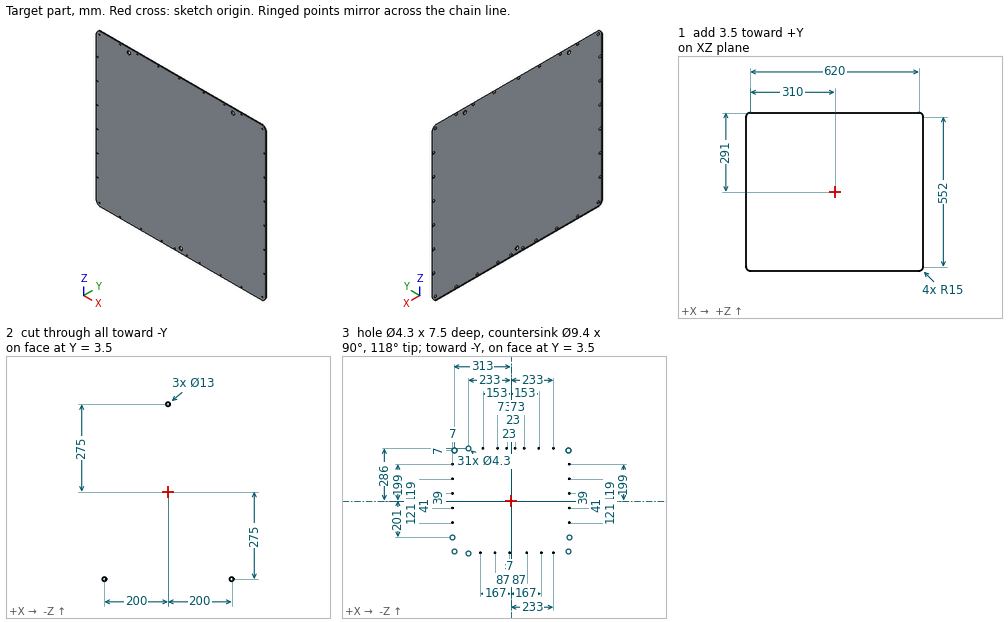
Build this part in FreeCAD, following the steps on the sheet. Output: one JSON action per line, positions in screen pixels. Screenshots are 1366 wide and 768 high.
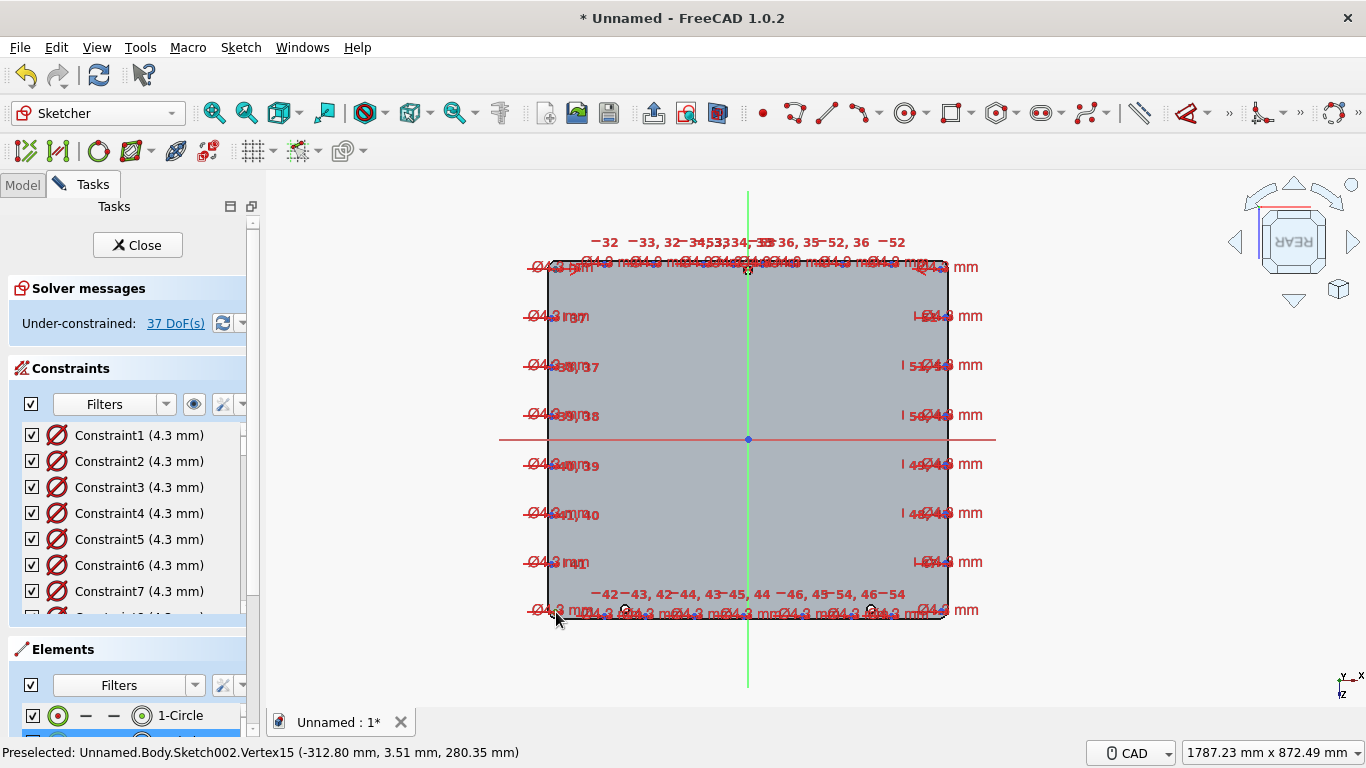
{"action": "left_click", "coordinate": [618, 440]}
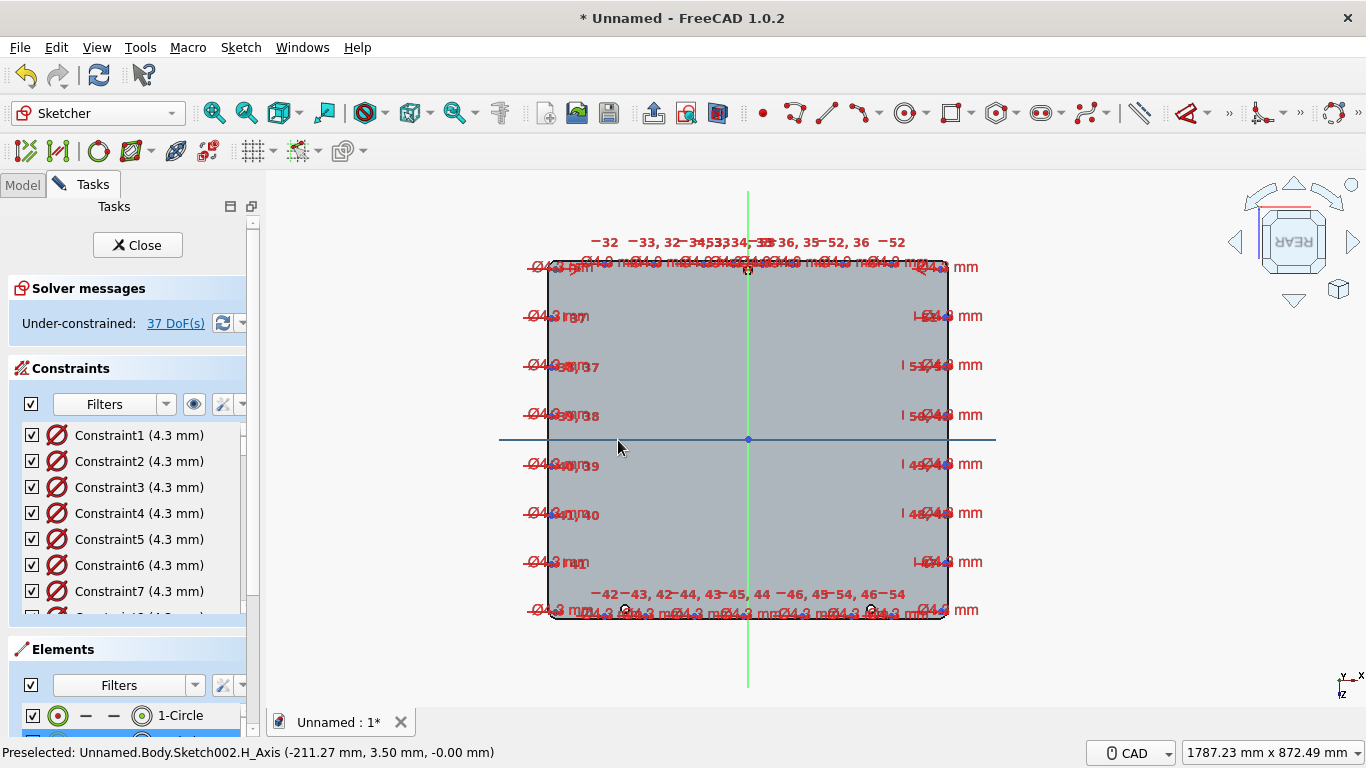
{"action": "key", "text": "s"}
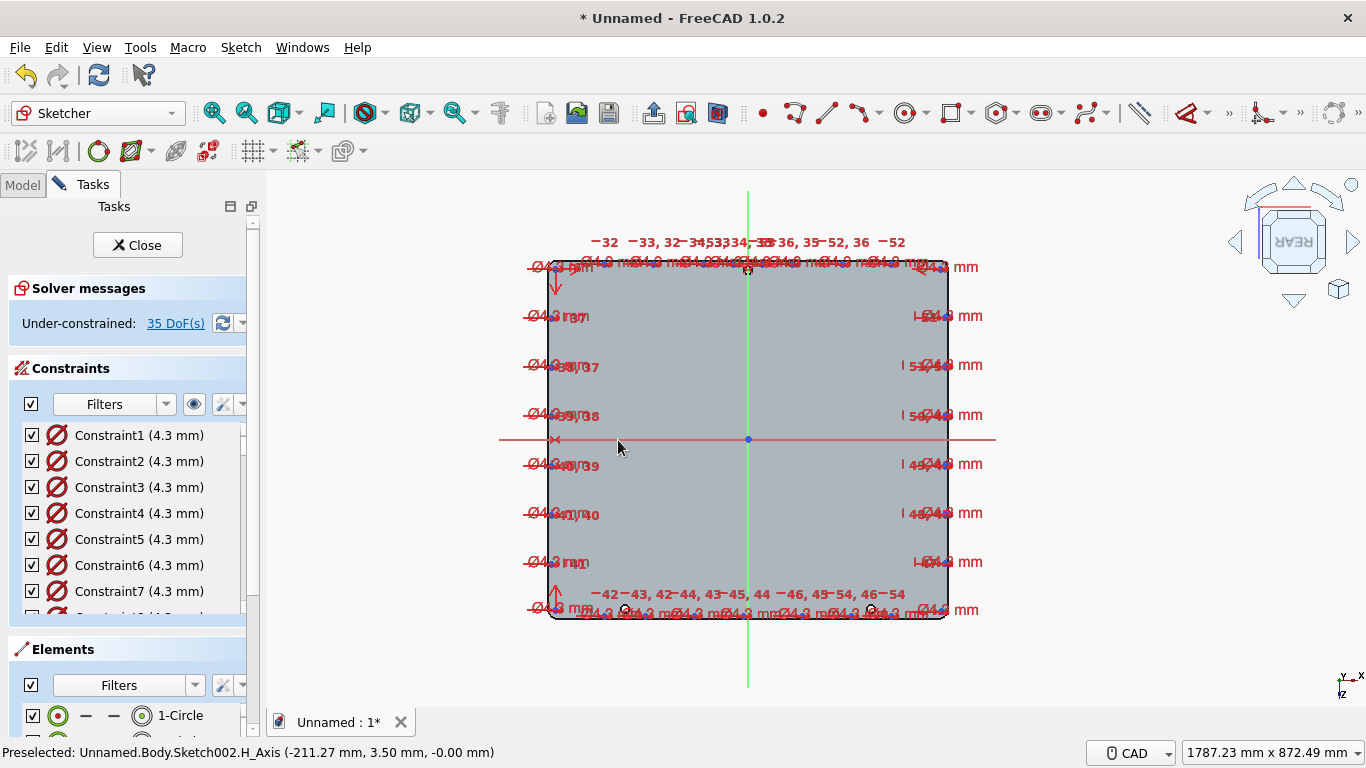
{"action": "left_click", "coordinate": [605, 264]}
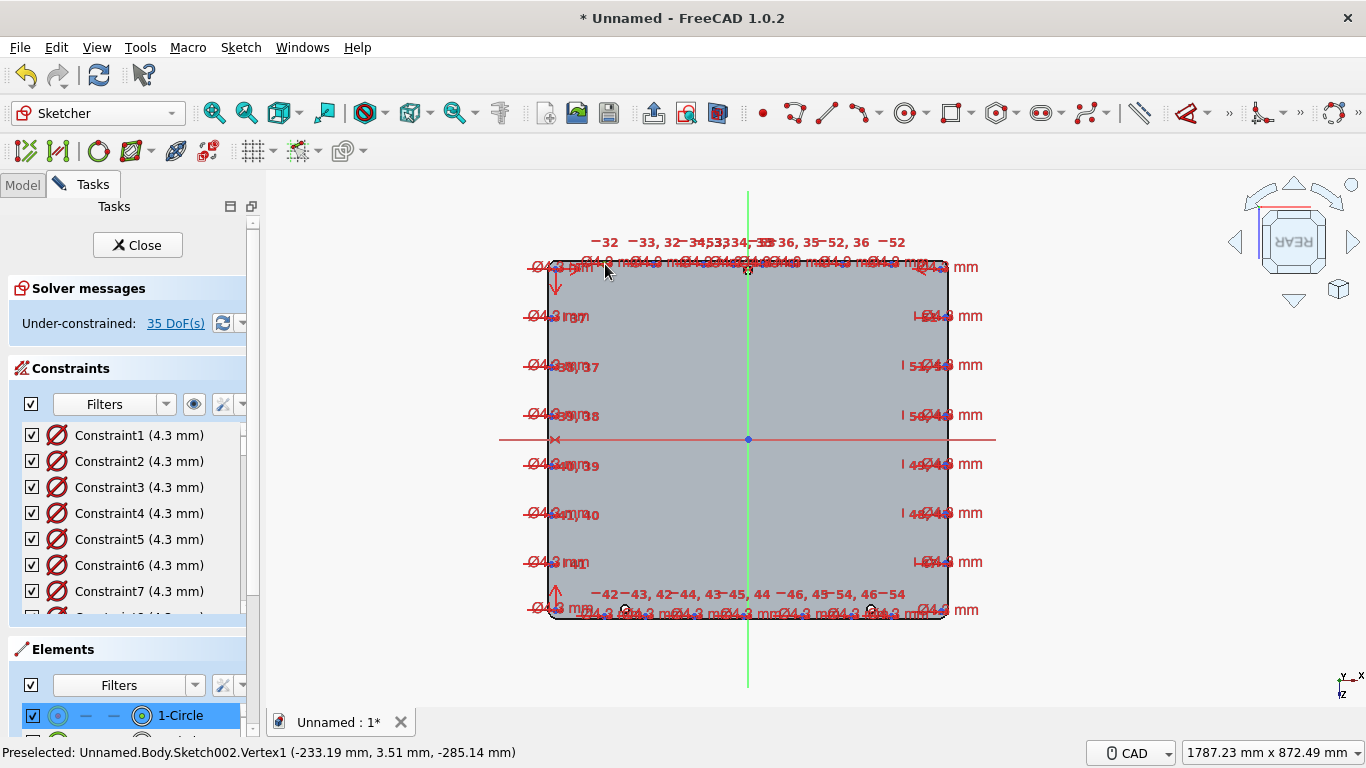
{"action": "left_click", "coordinate": [605, 616]}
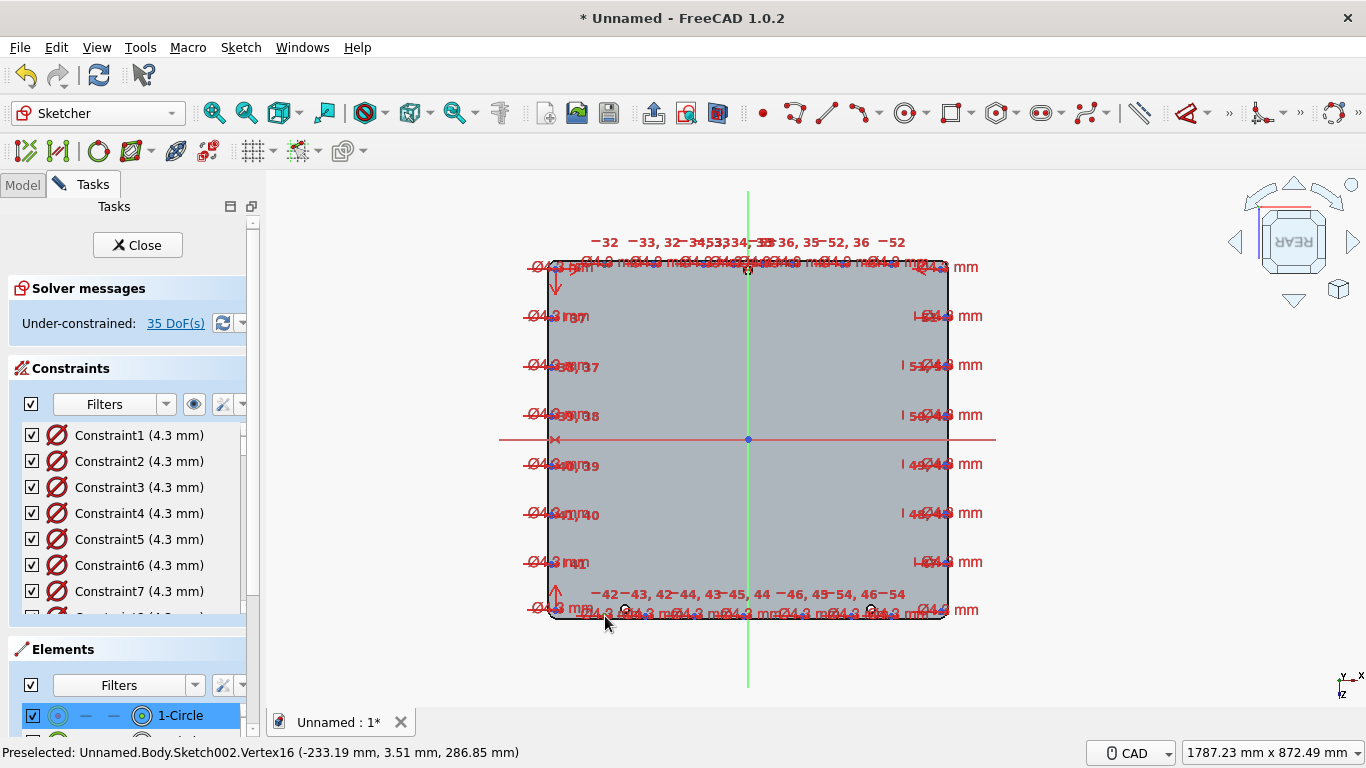
{"action": "left_click", "coordinate": [618, 440]}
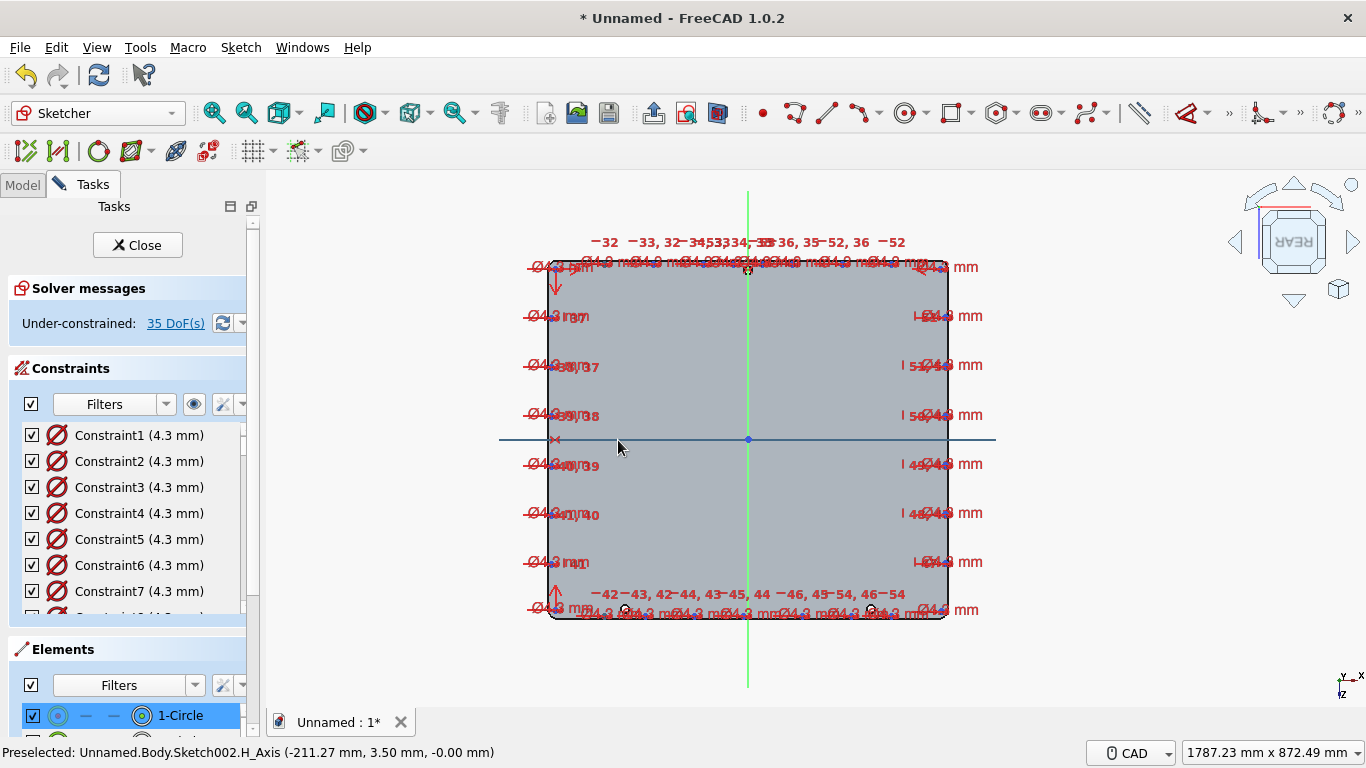
{"action": "key", "text": "s"}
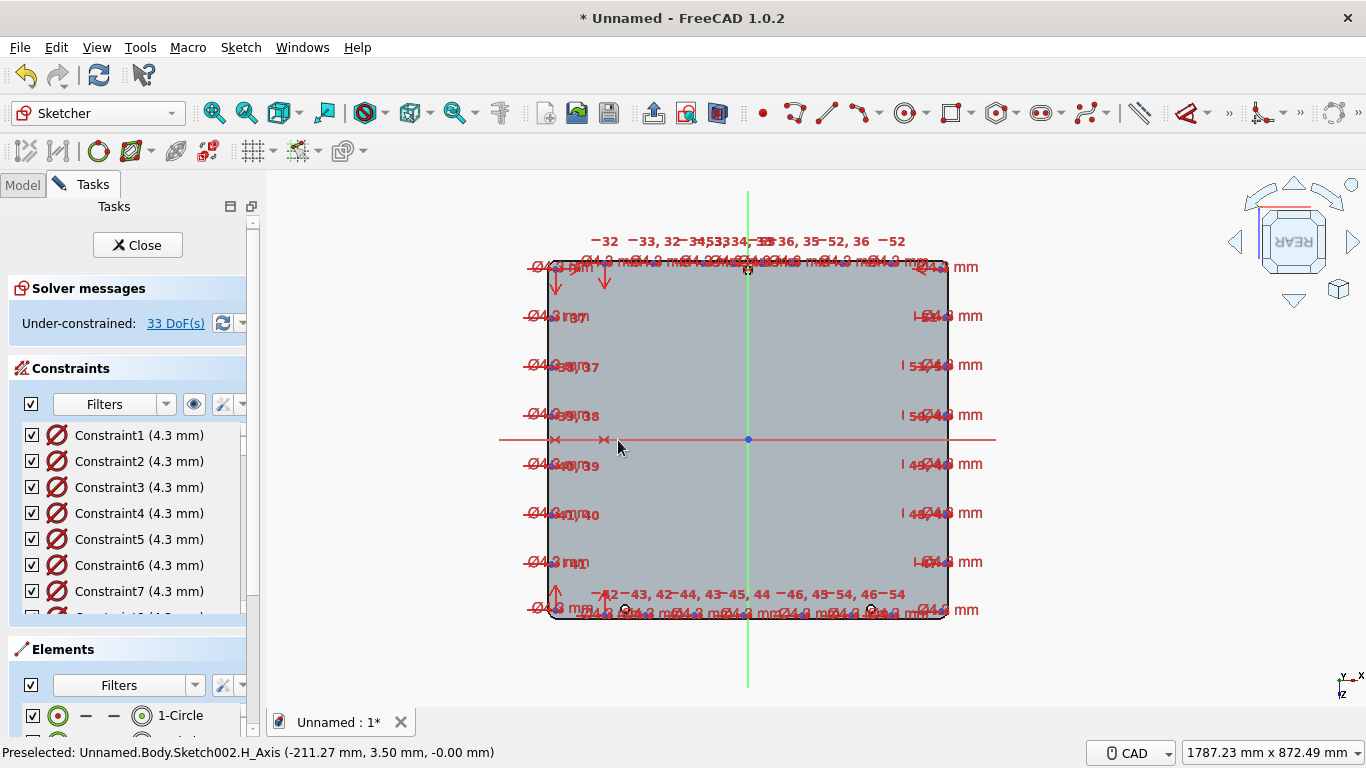
{"action": "left_click", "coordinate": [941, 269]}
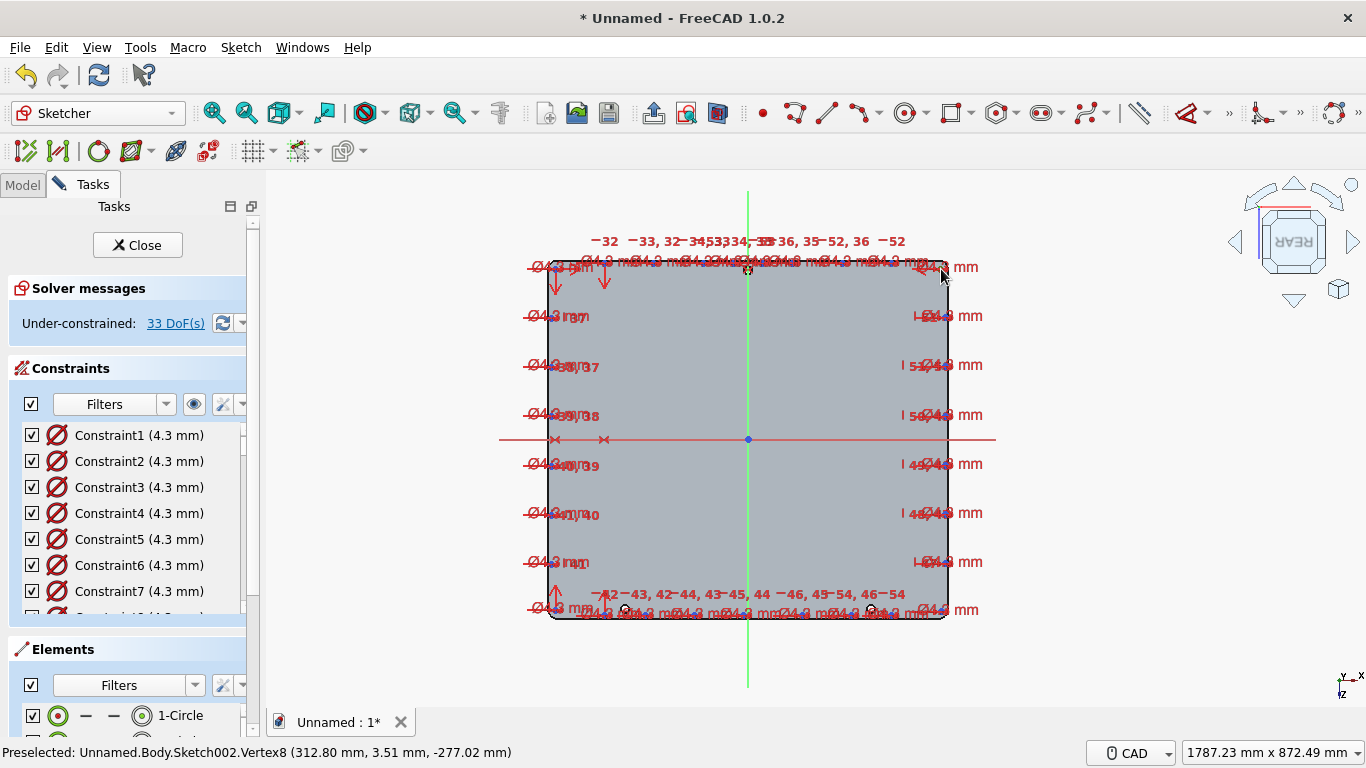
{"action": "left_click", "coordinate": [941, 612]}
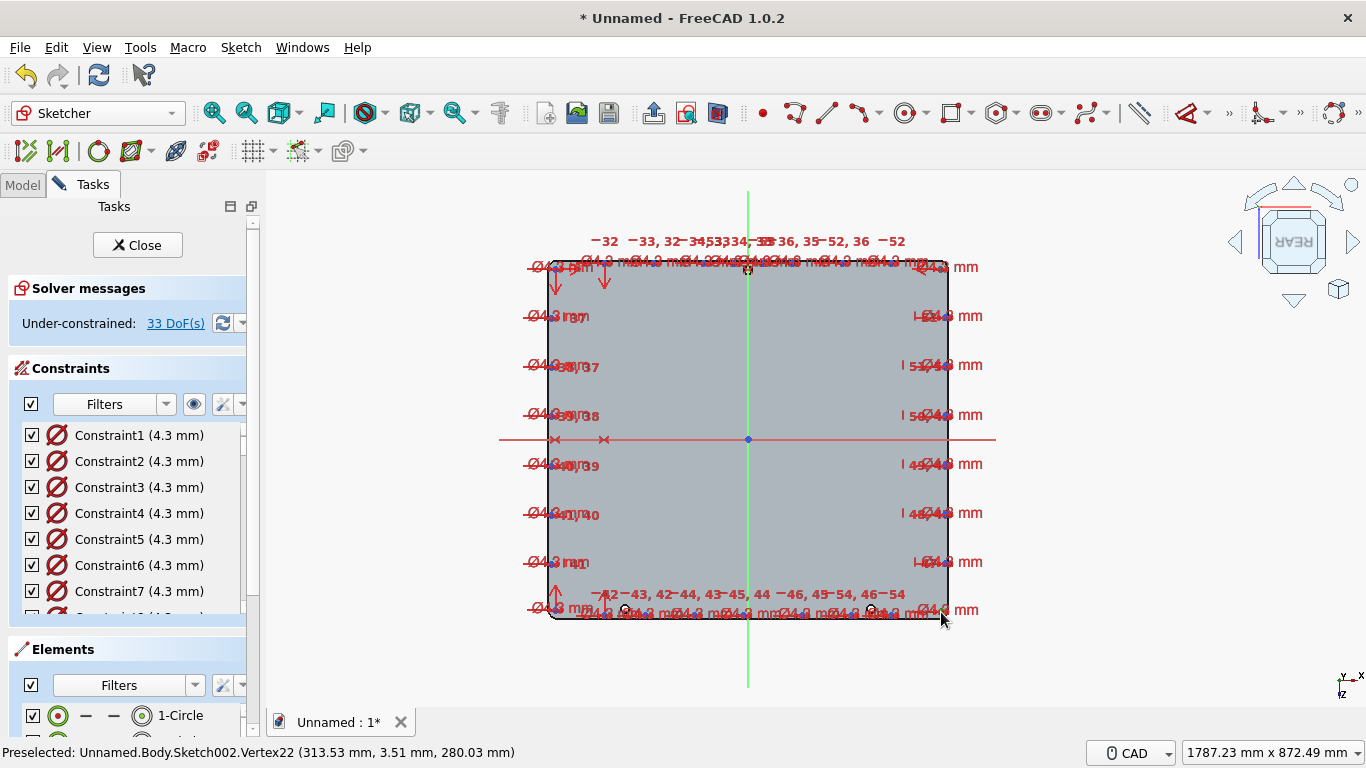
{"action": "left_click", "coordinate": [618, 440]}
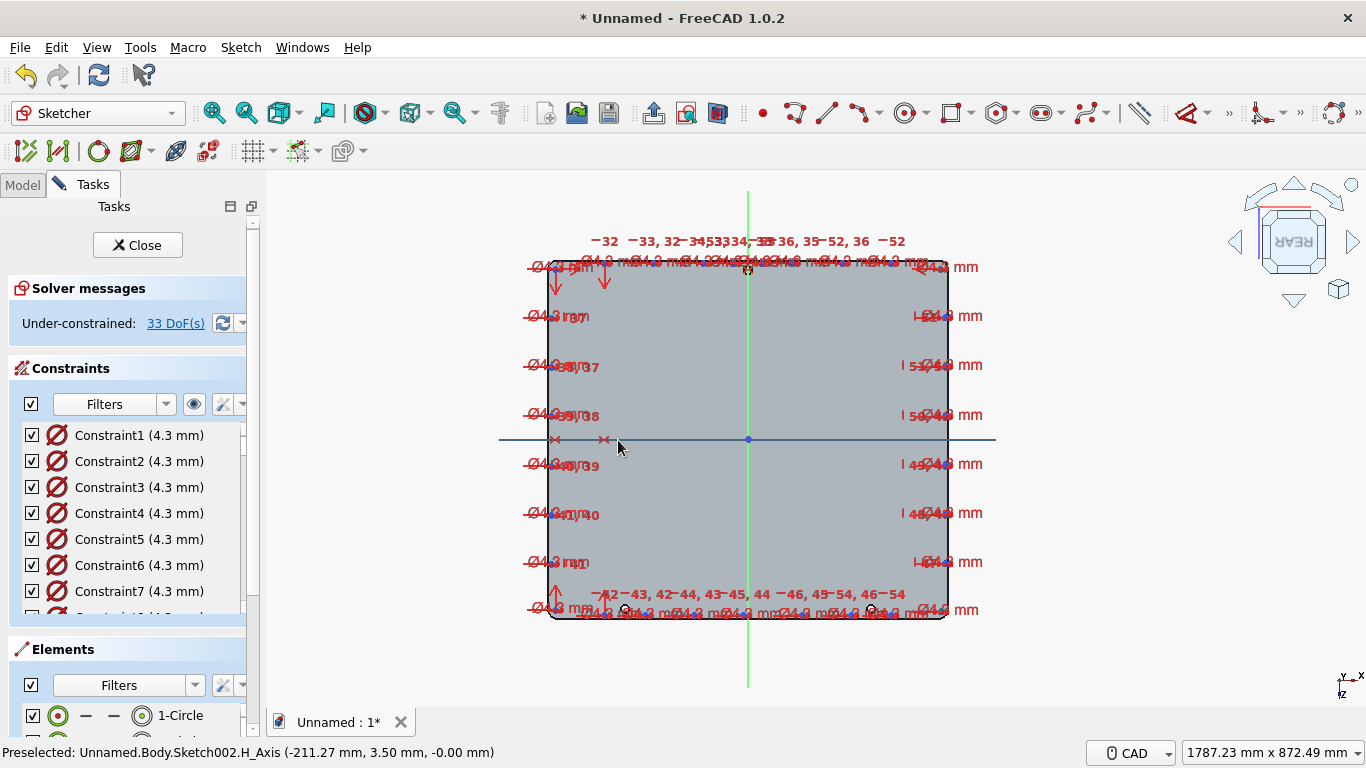
{"action": "key", "text": "s"}